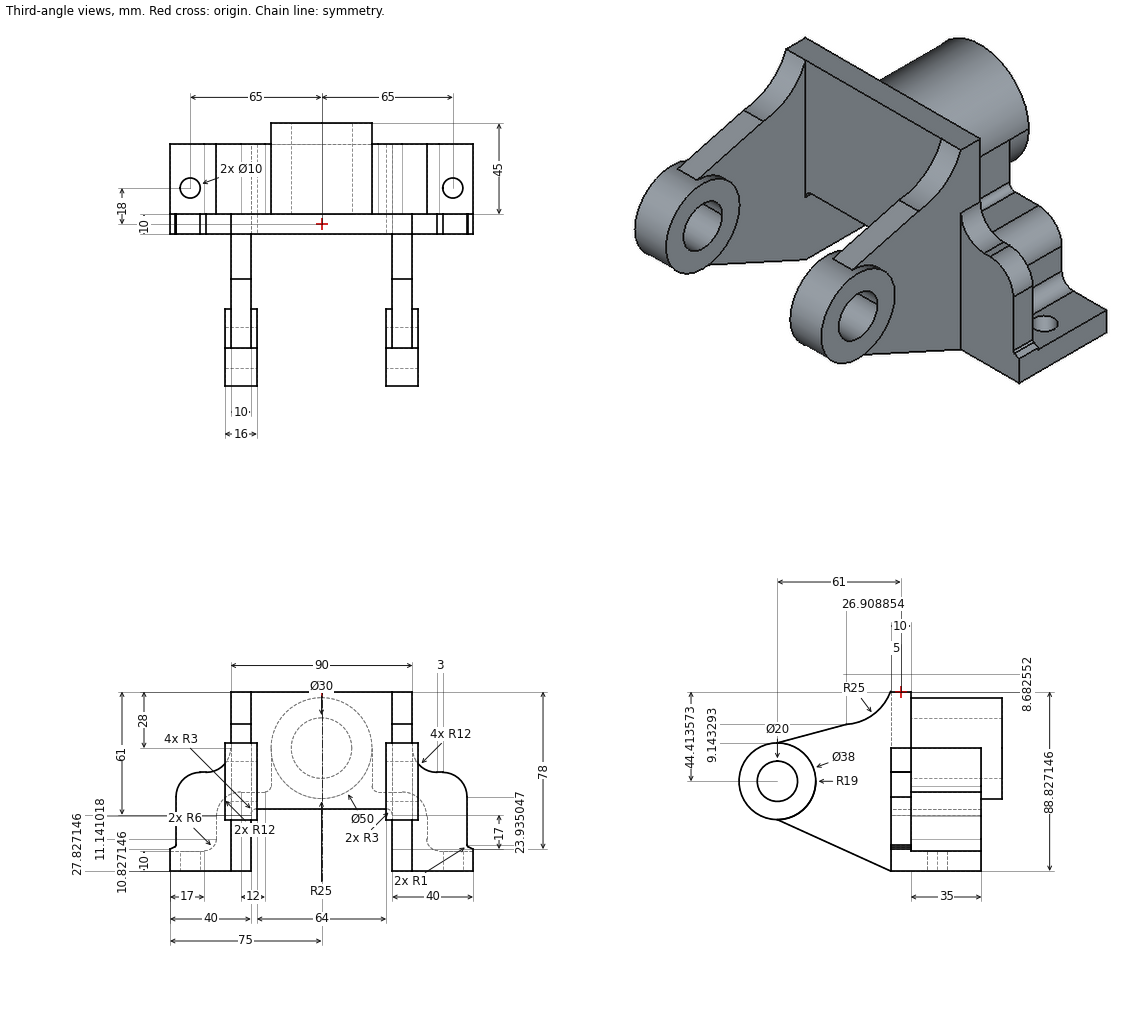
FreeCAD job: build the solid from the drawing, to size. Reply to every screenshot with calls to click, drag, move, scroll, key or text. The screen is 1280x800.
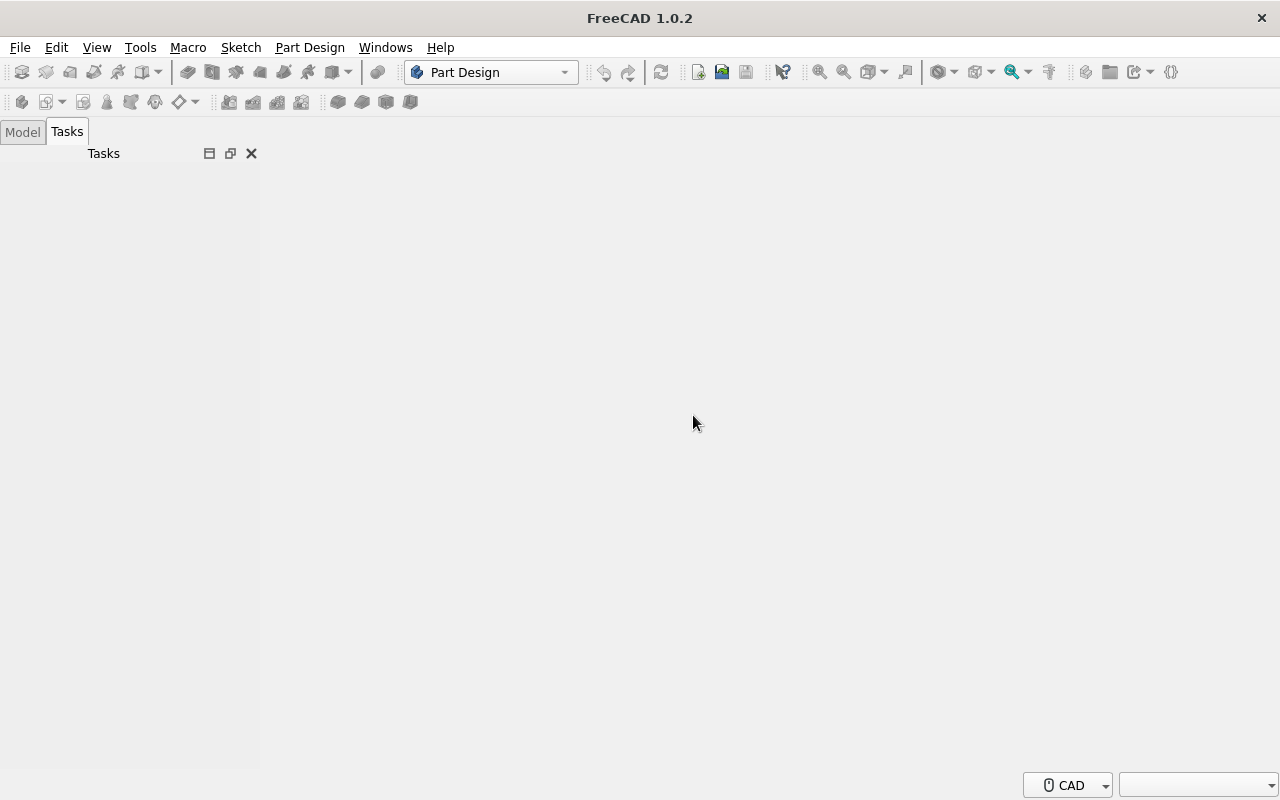
key(ctrl+n)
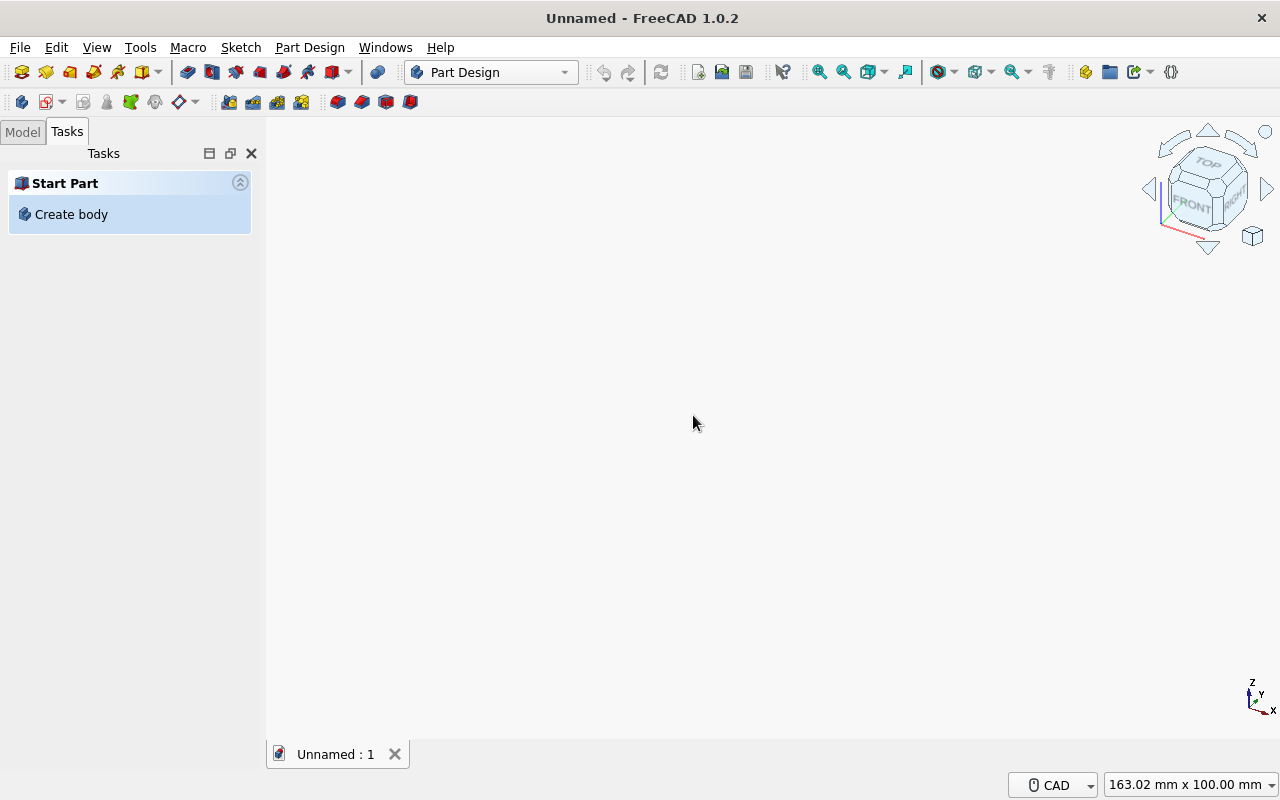
click(46, 102)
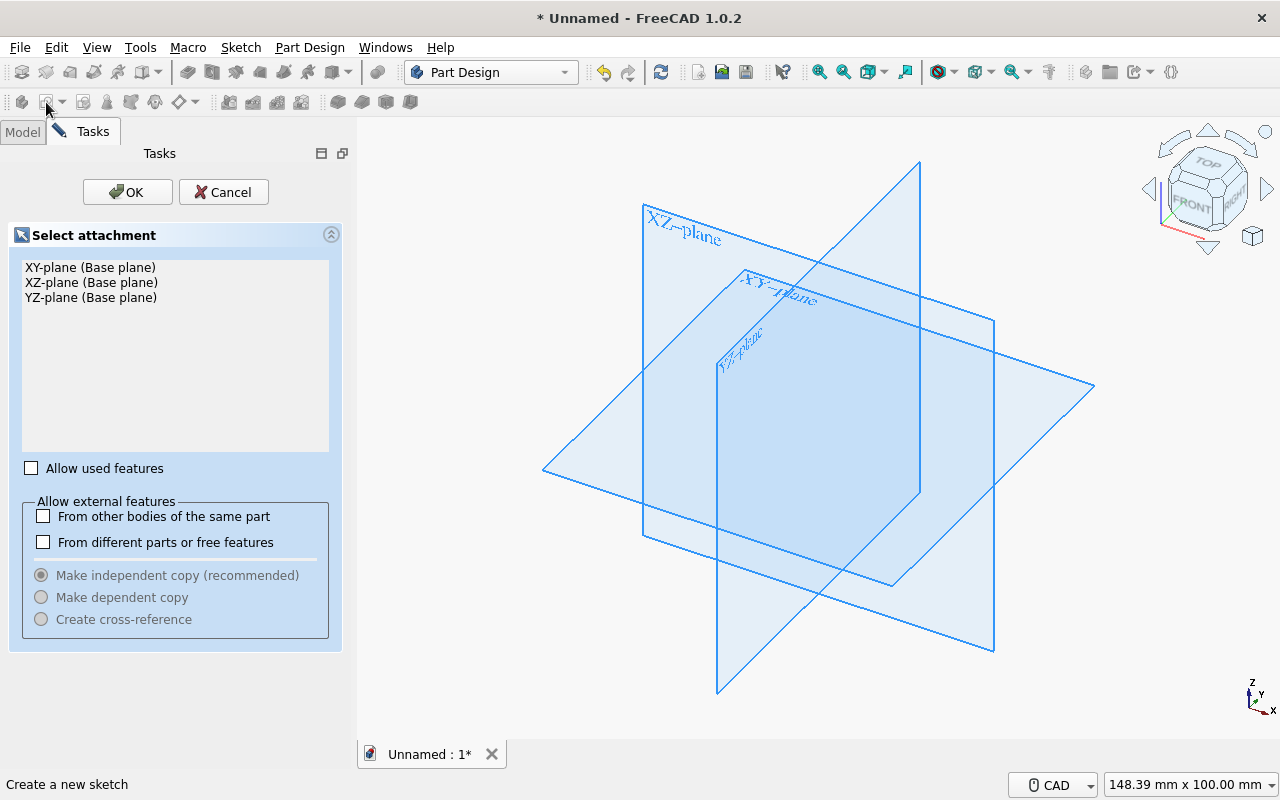
click(82, 282)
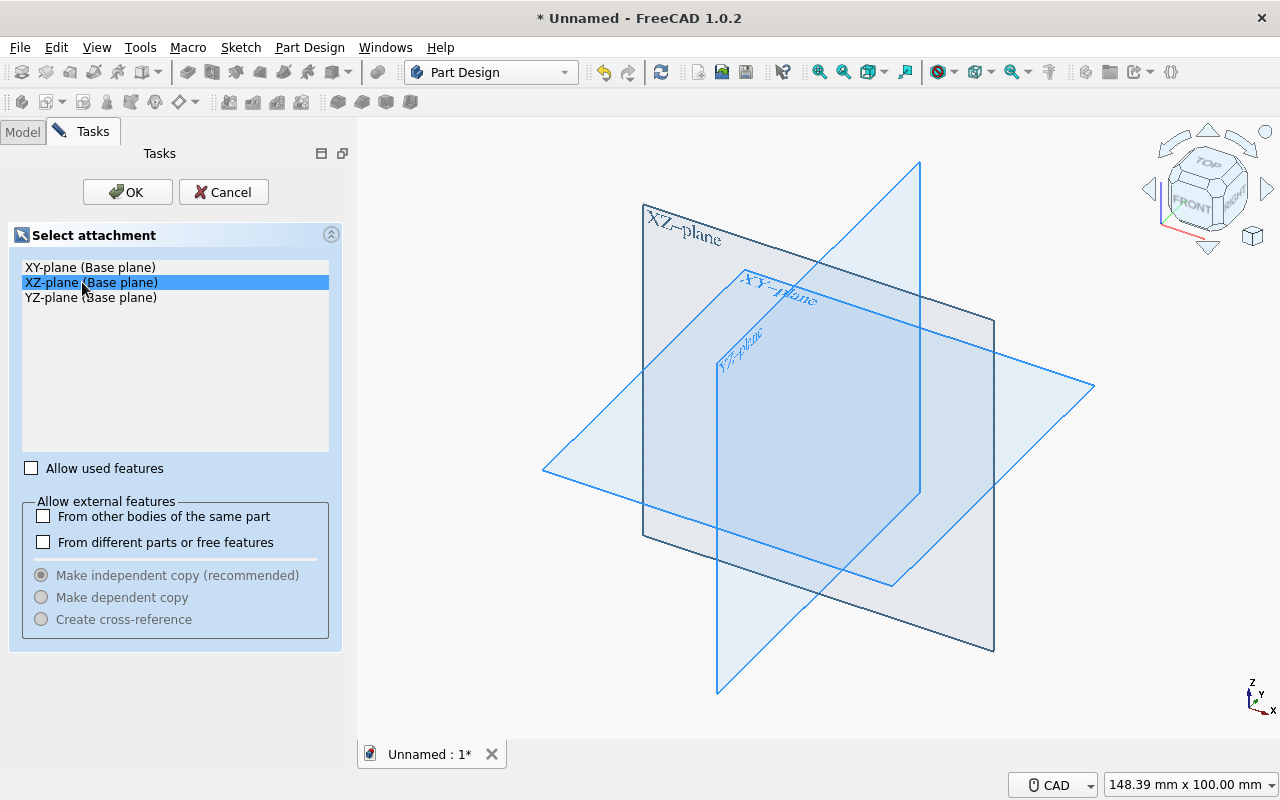
click(128, 192)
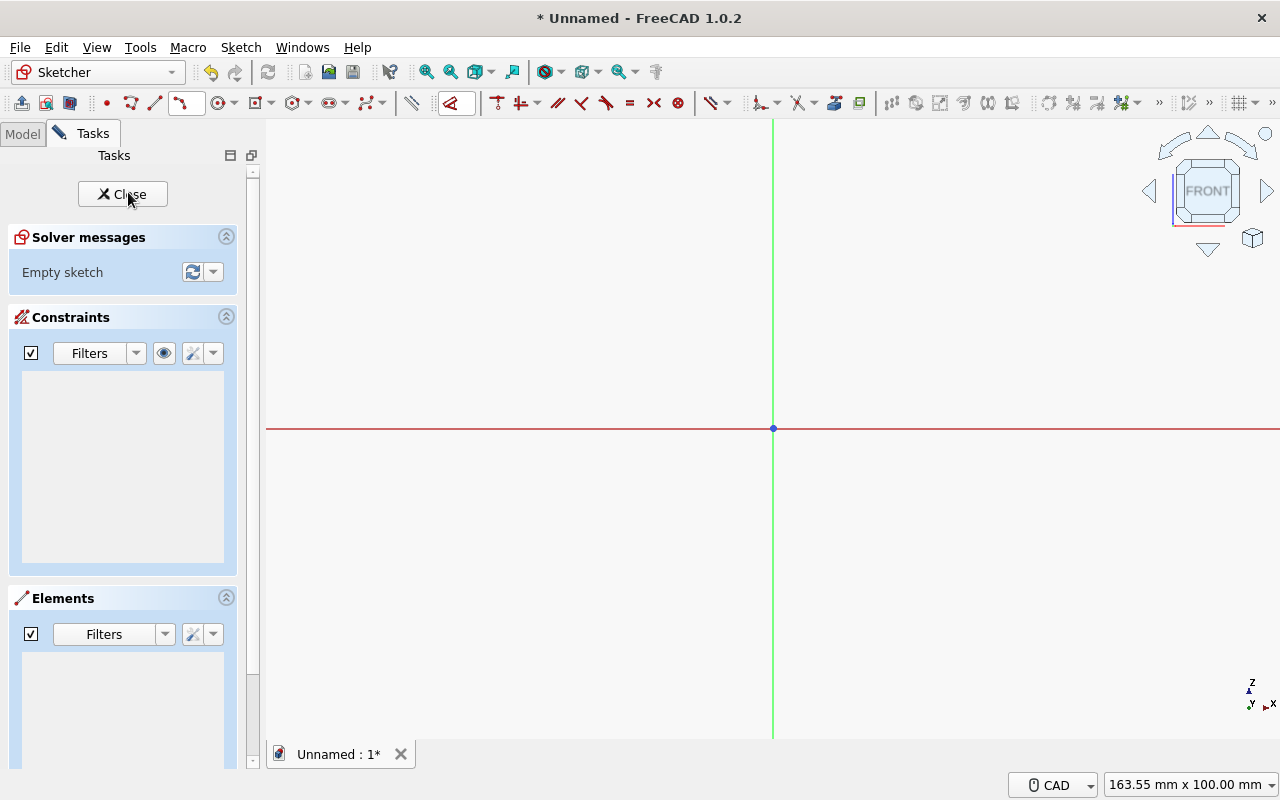
scroll(565, 147, down, 2)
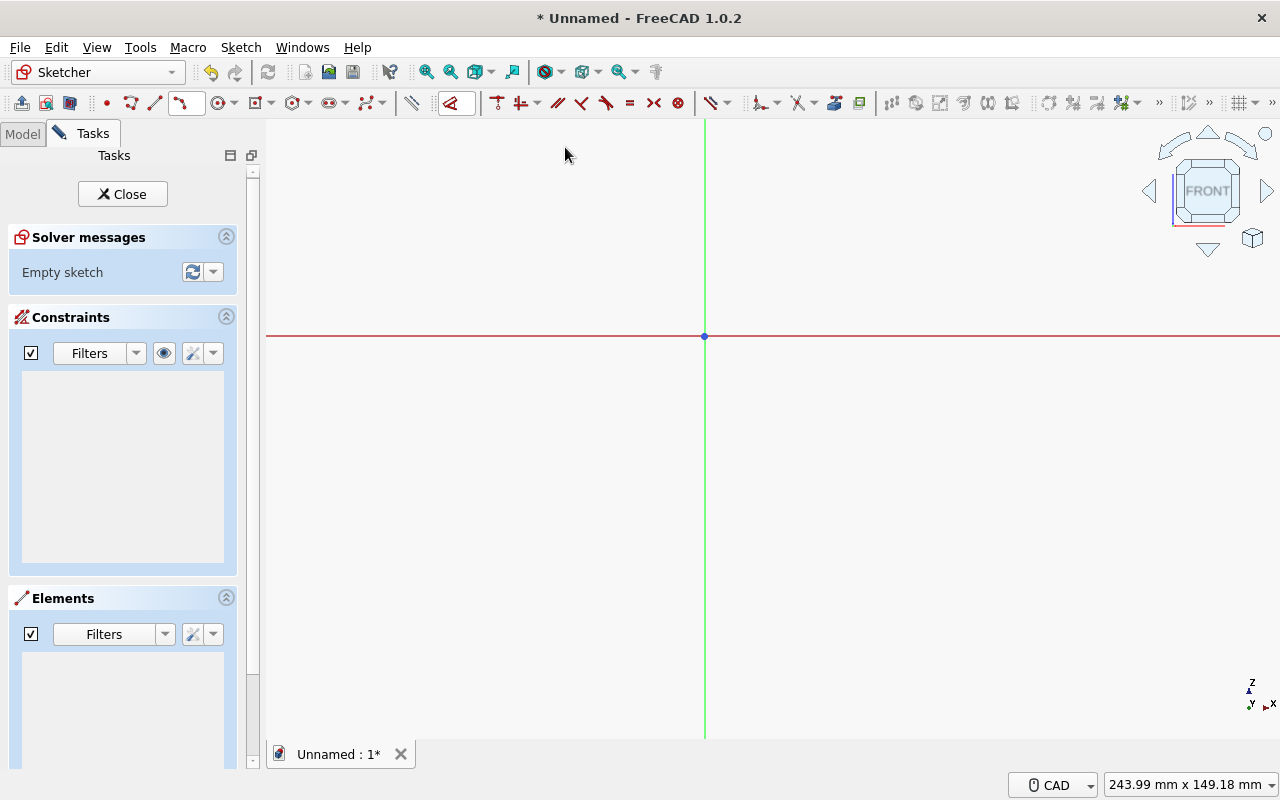
key(g)
key(l)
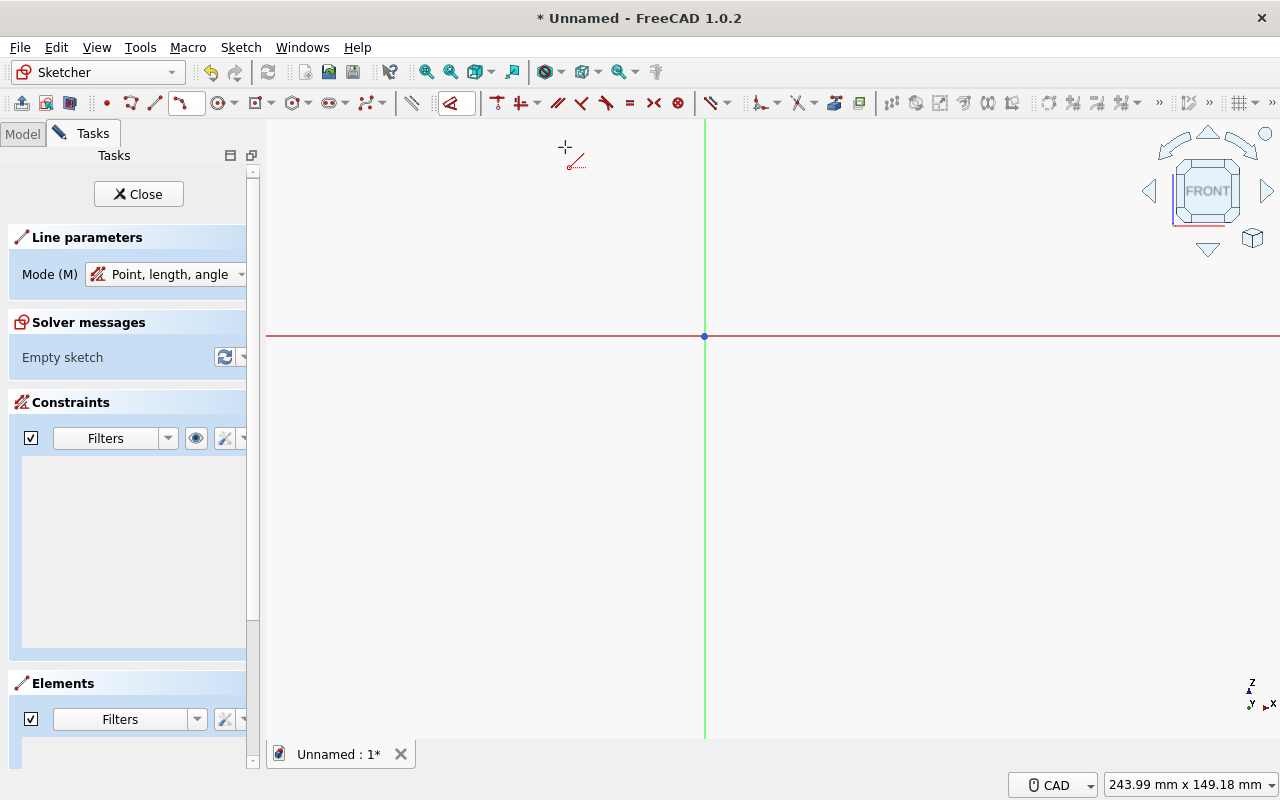
click(941, 502)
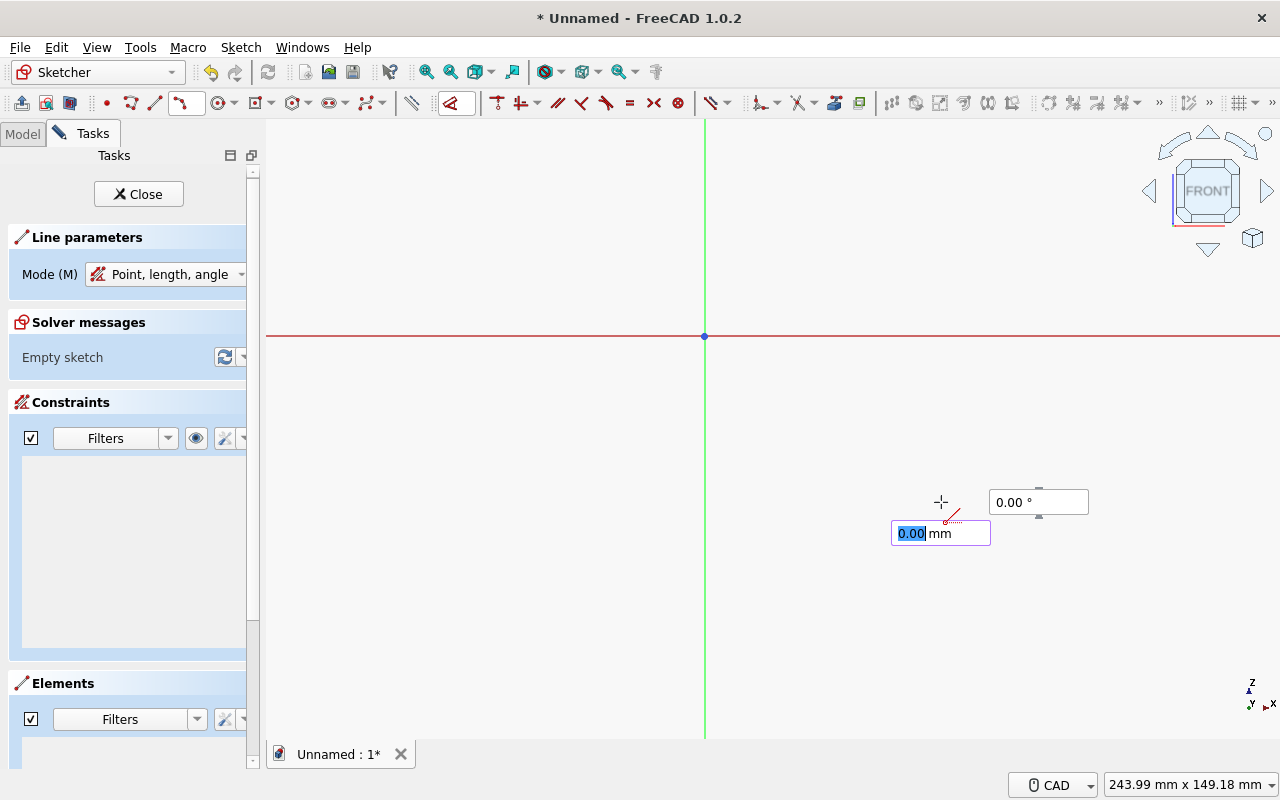
scroll(954, 502, up, 2)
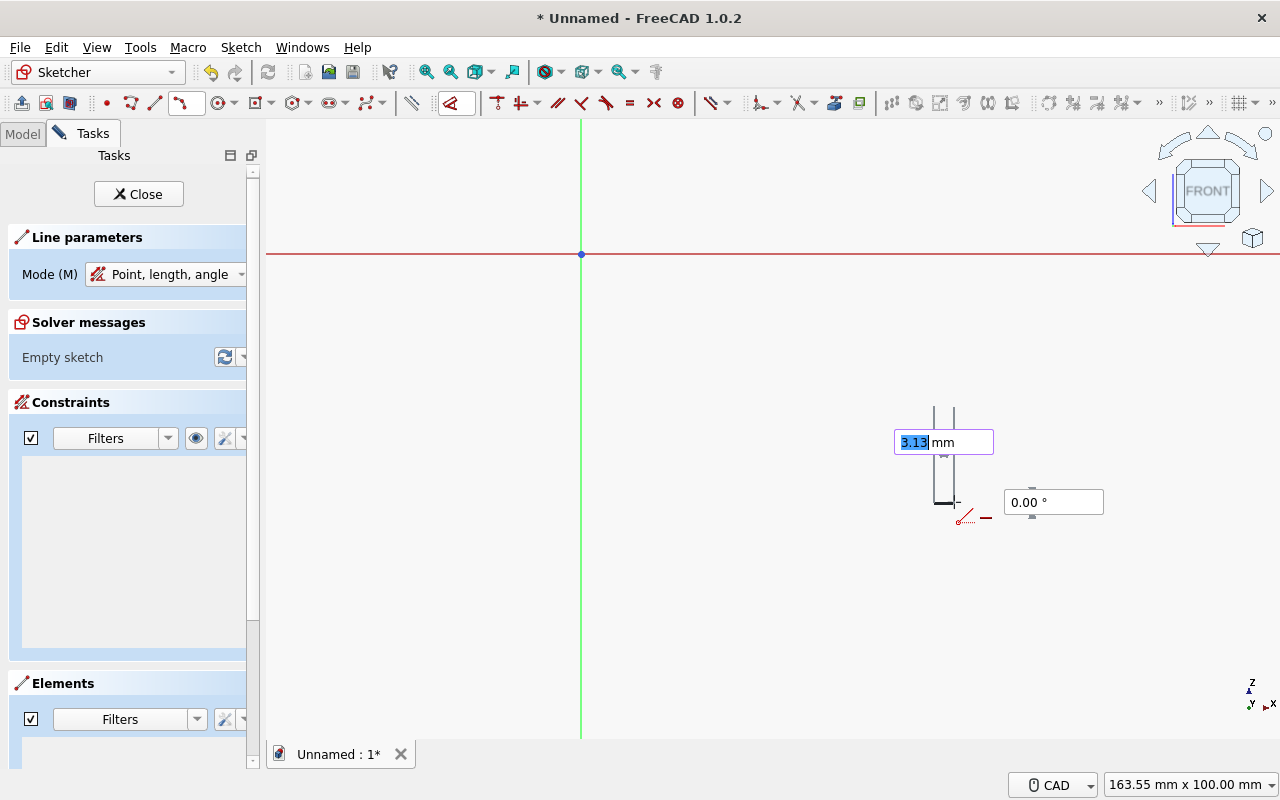
click(953, 502)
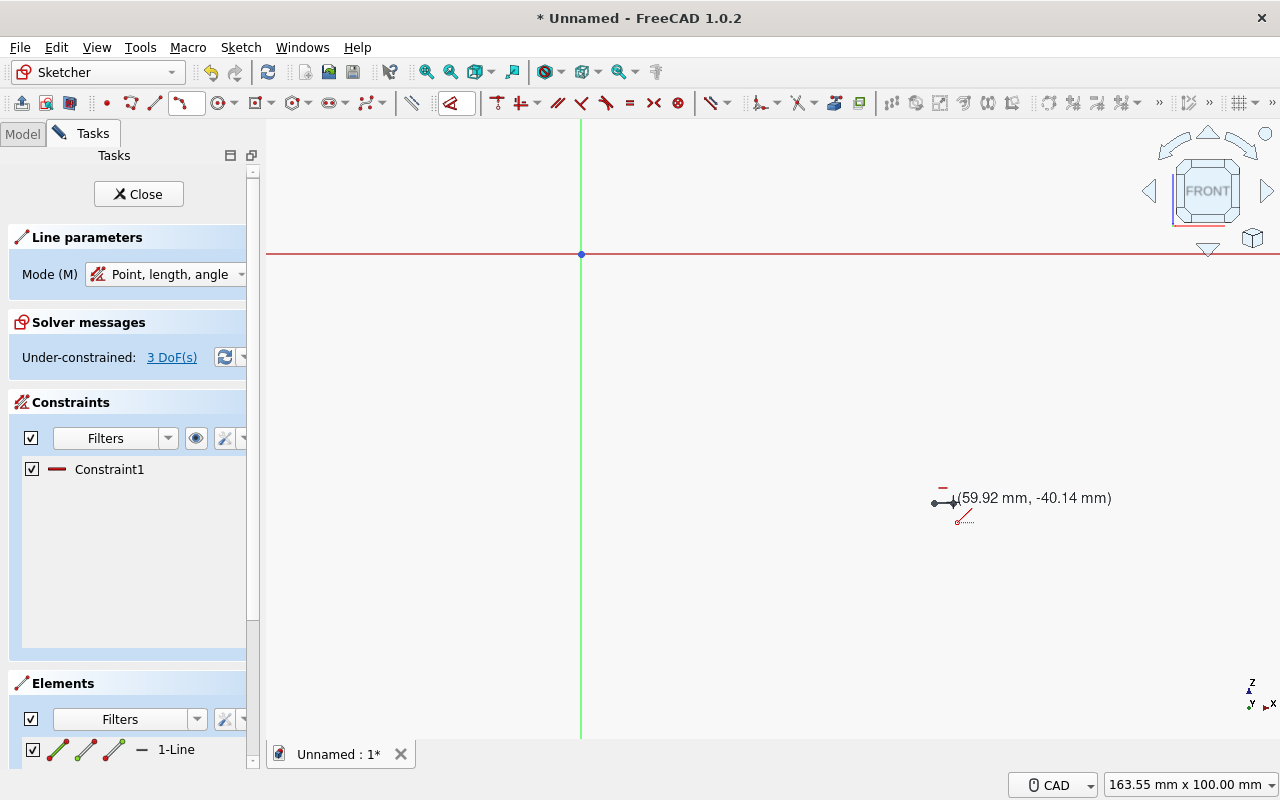
click(1028, 577)